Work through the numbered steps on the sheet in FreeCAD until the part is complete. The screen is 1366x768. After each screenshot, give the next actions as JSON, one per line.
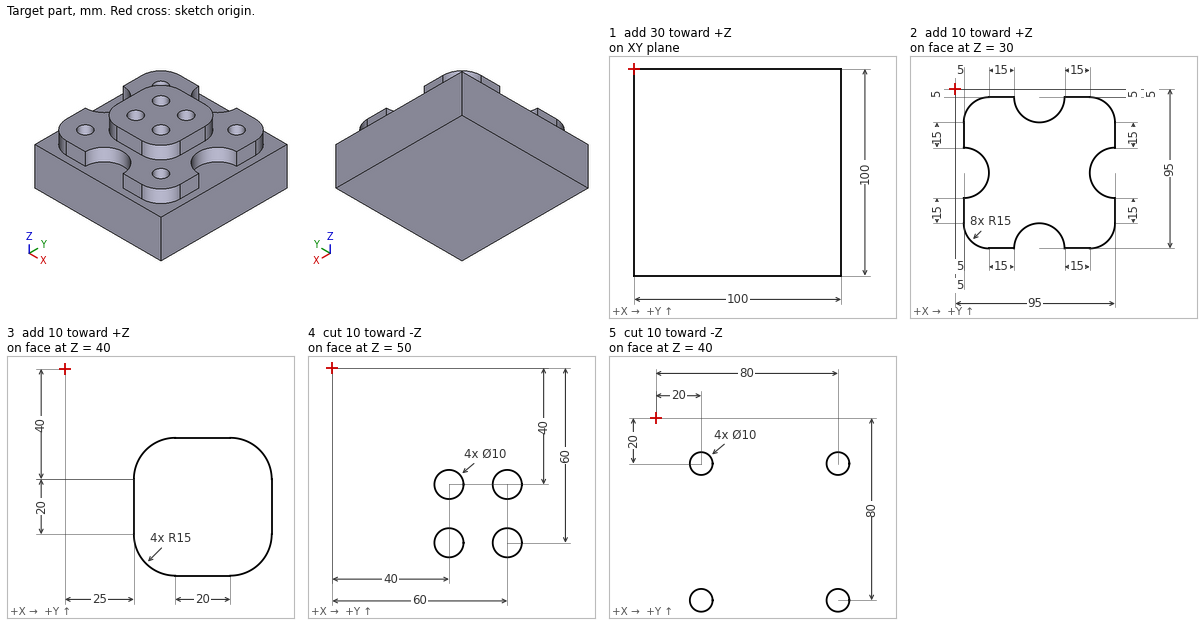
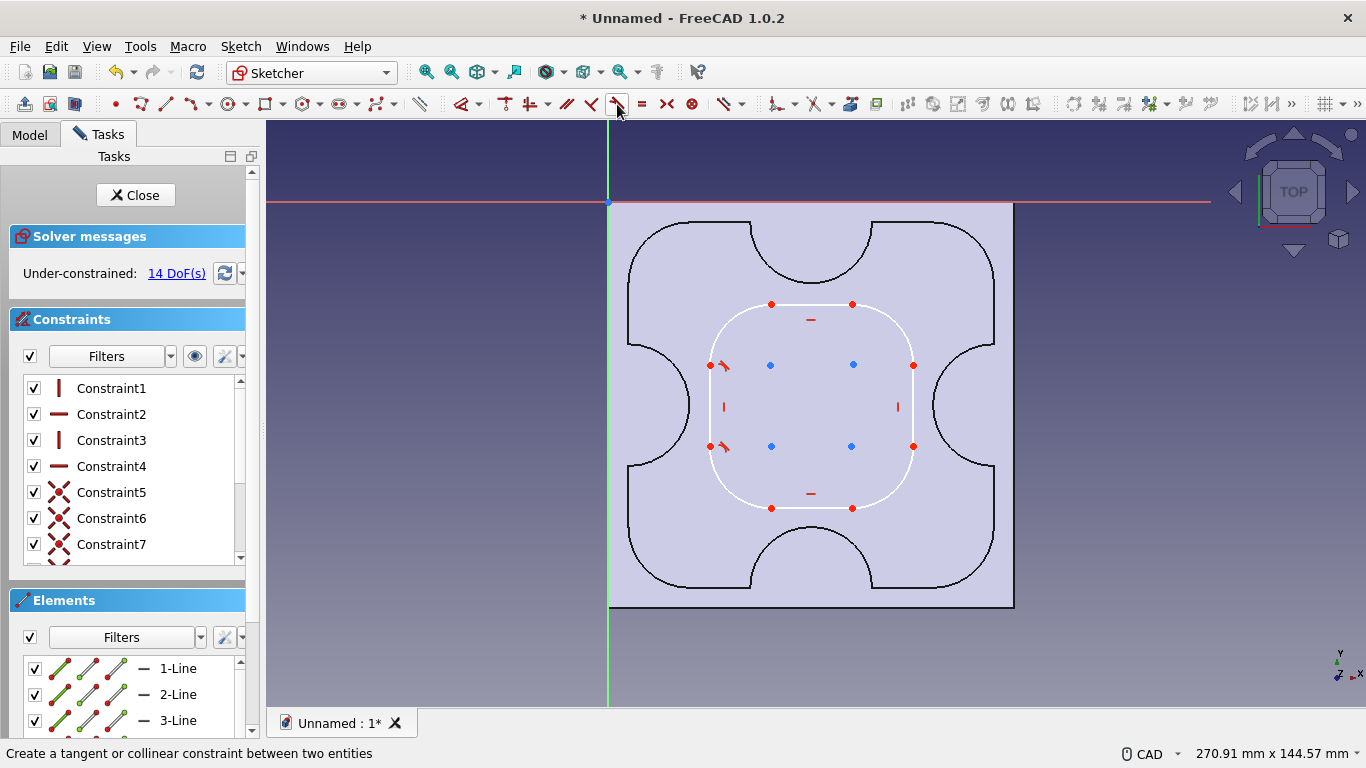
{"action": "left_click", "coordinate": [795, 508]}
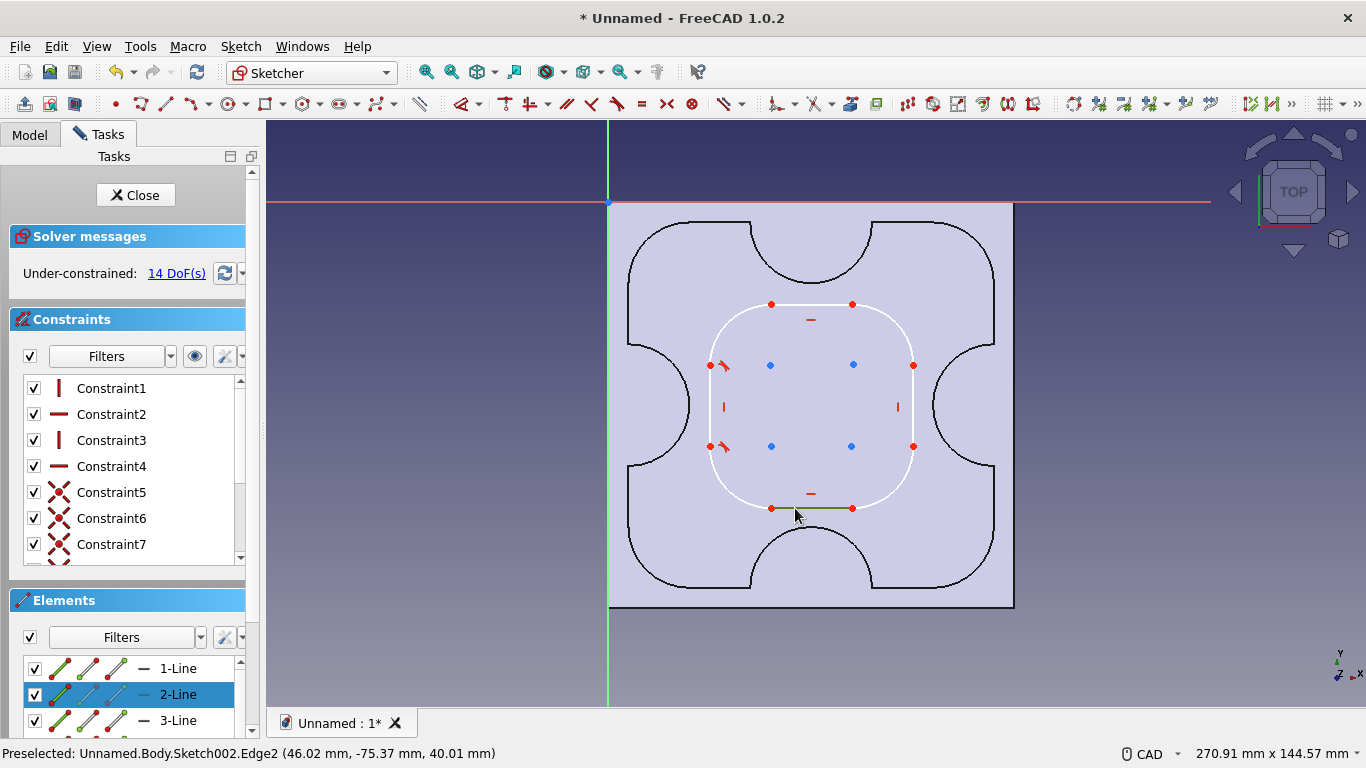
{"action": "left_click", "coordinate": [717, 474]}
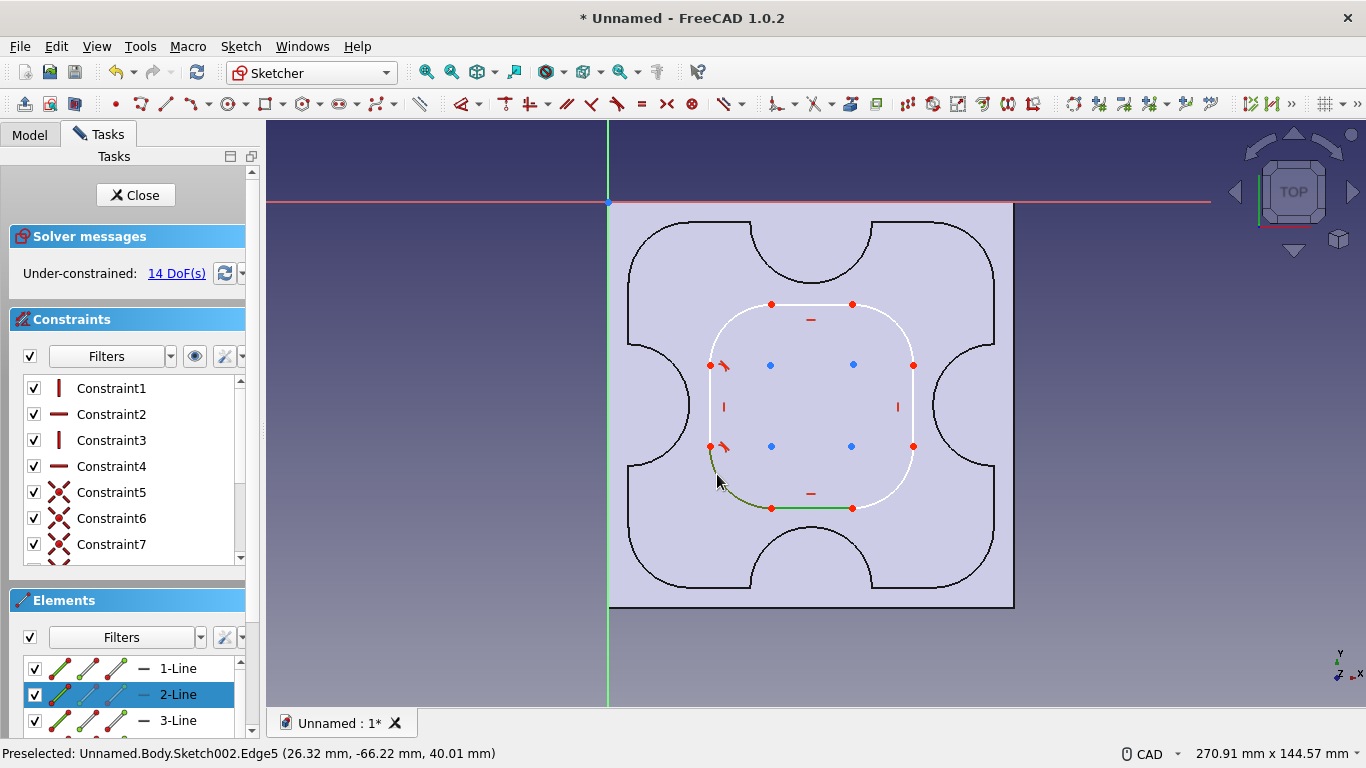
{"action": "key", "text": "t"}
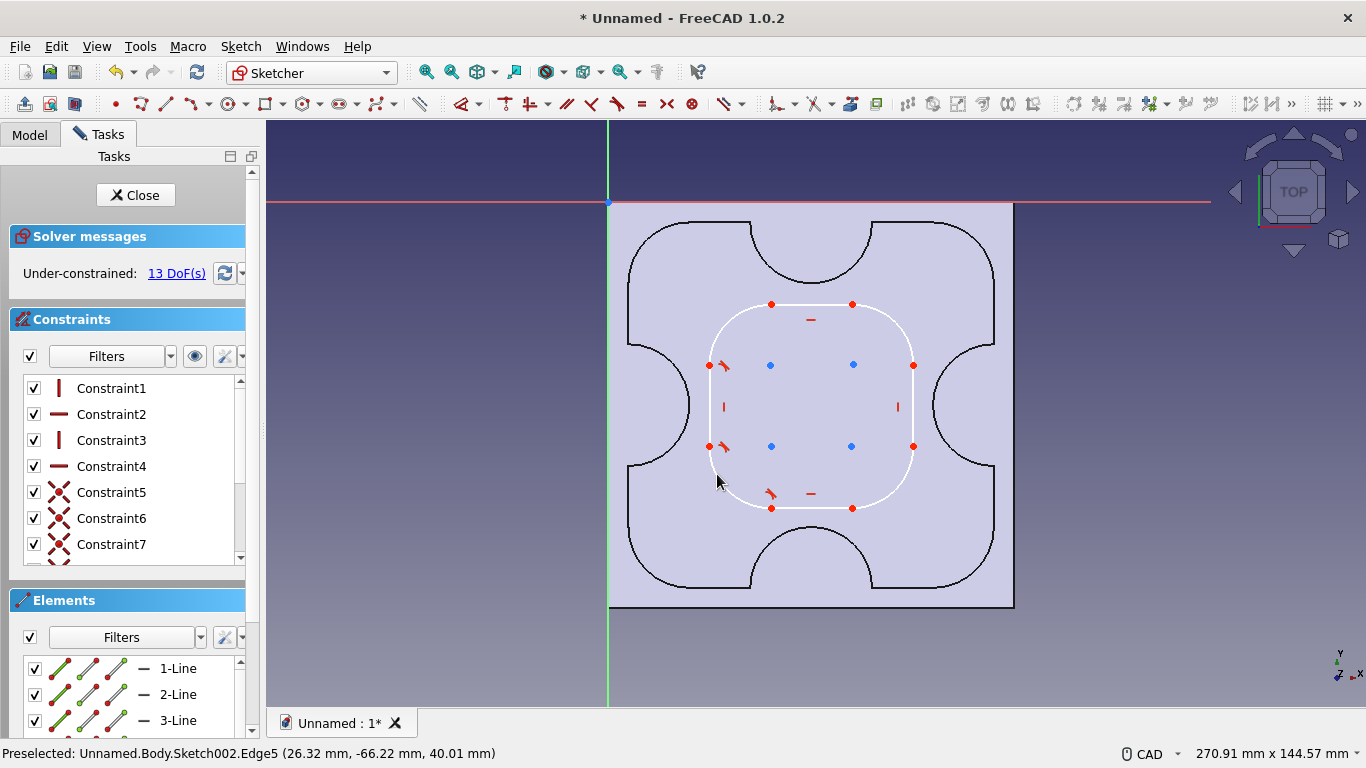
{"action": "left_click", "coordinate": [795, 508]}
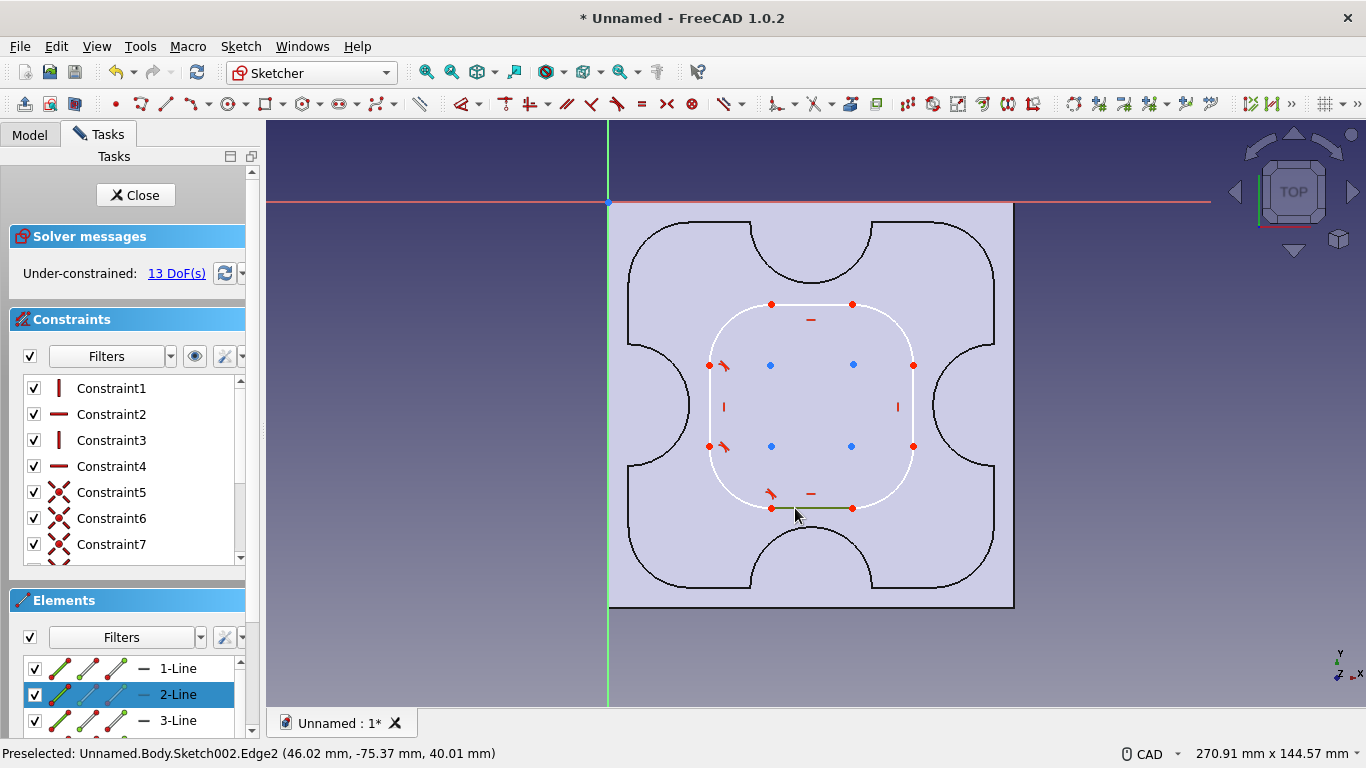
{"action": "left_click", "coordinate": [880, 501]}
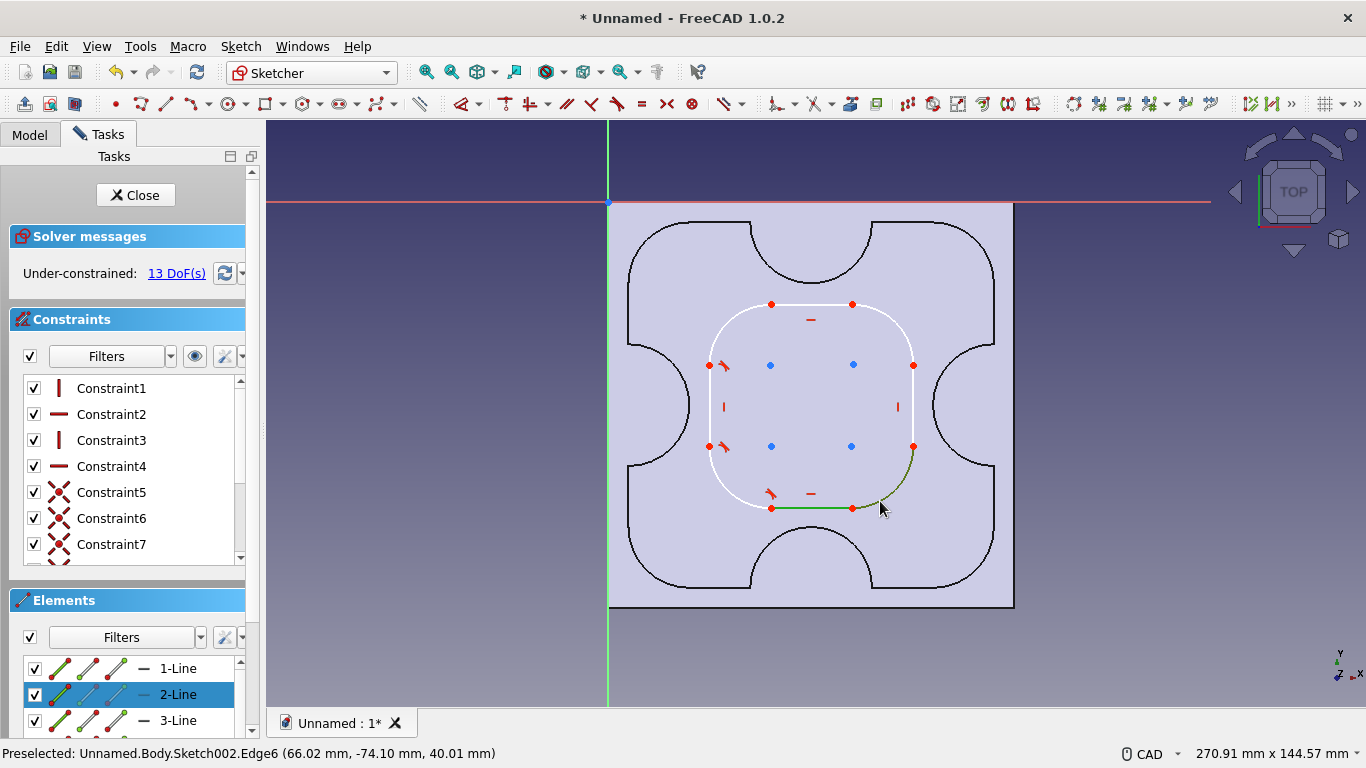
{"action": "left_click", "coordinate": [617, 104]}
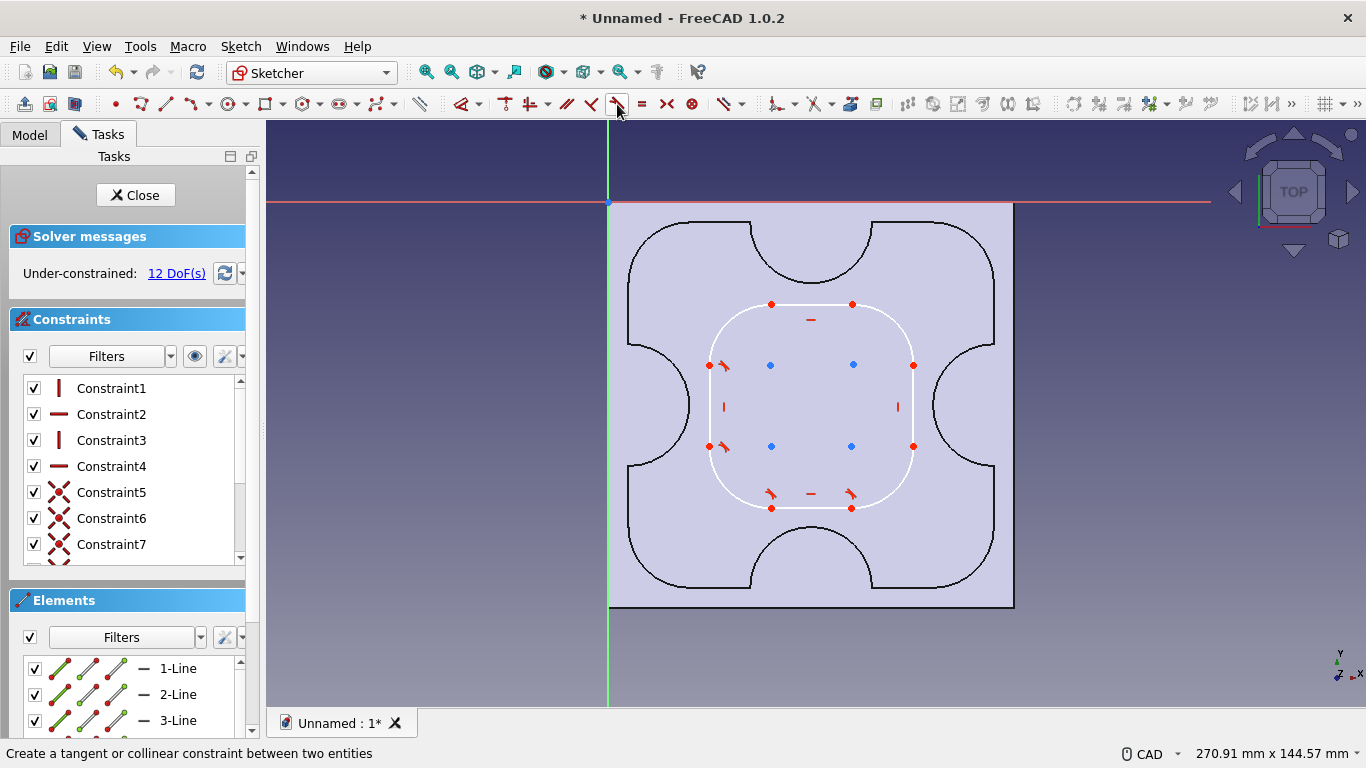
{"action": "left_click", "coordinate": [913, 423]}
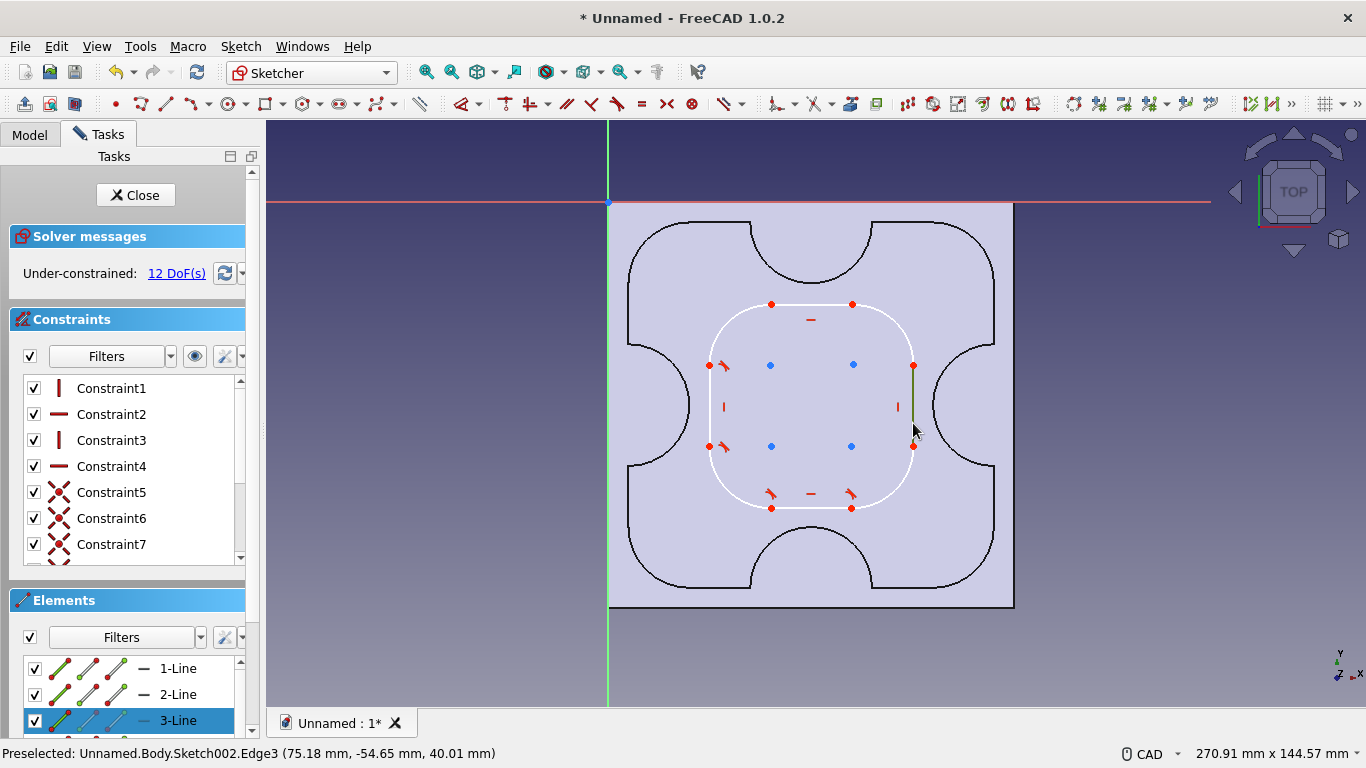
{"action": "left_click", "coordinate": [880, 502]}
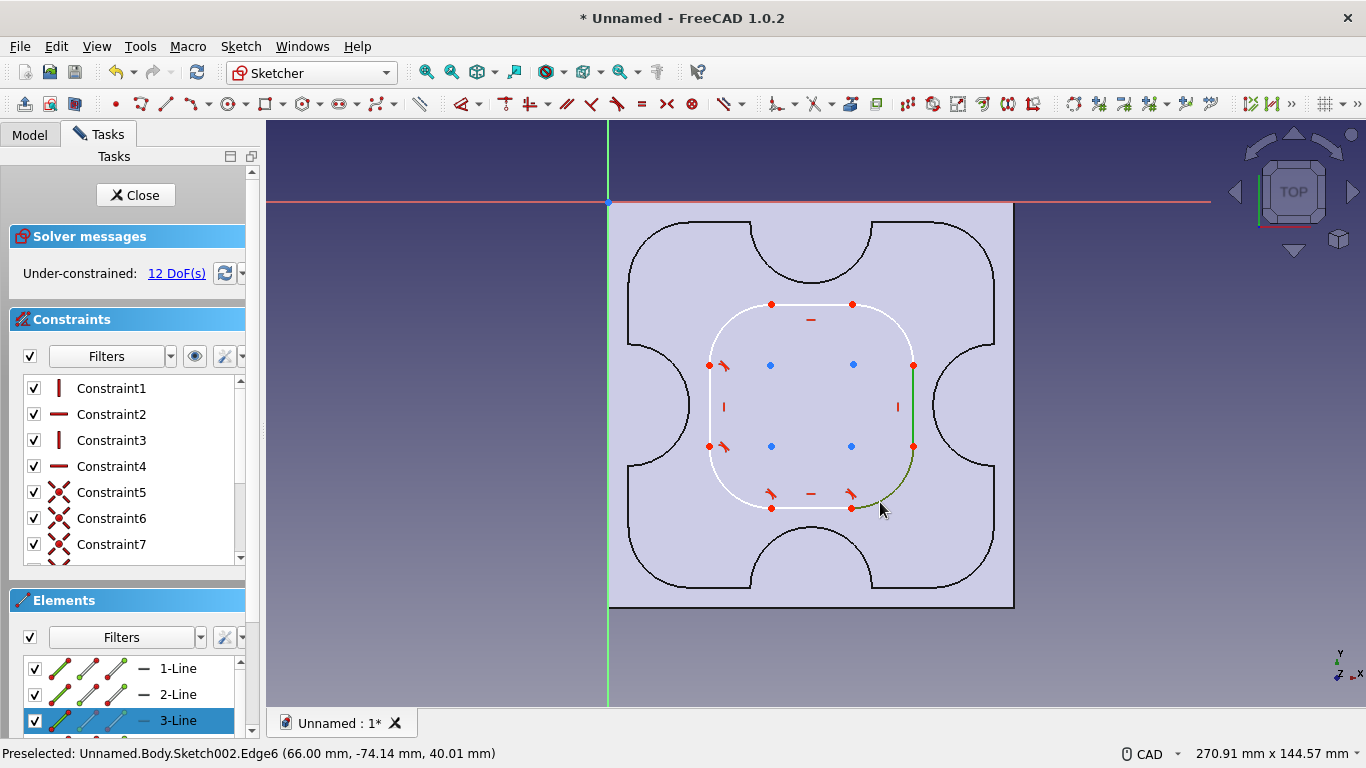
{"action": "left_click", "coordinate": [617, 104]}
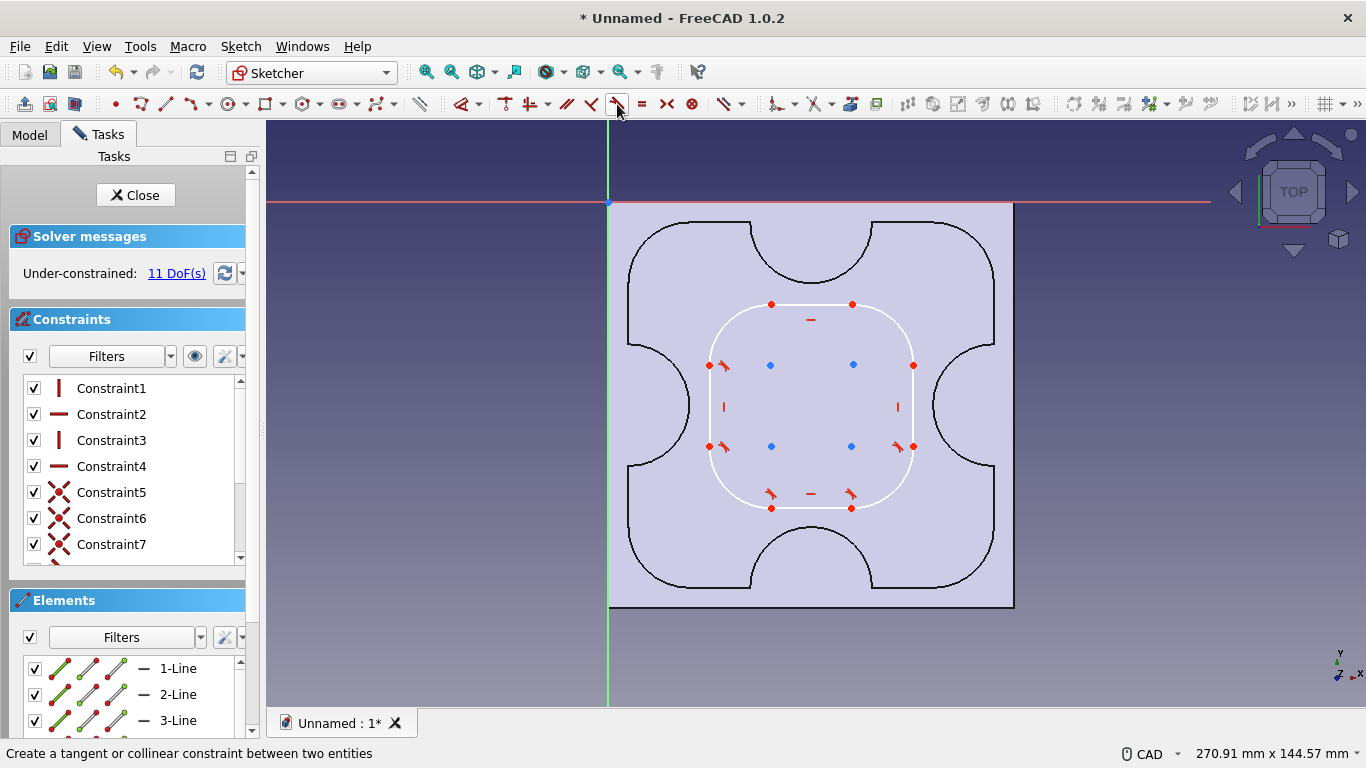
{"action": "left_click", "coordinate": [913, 422]}